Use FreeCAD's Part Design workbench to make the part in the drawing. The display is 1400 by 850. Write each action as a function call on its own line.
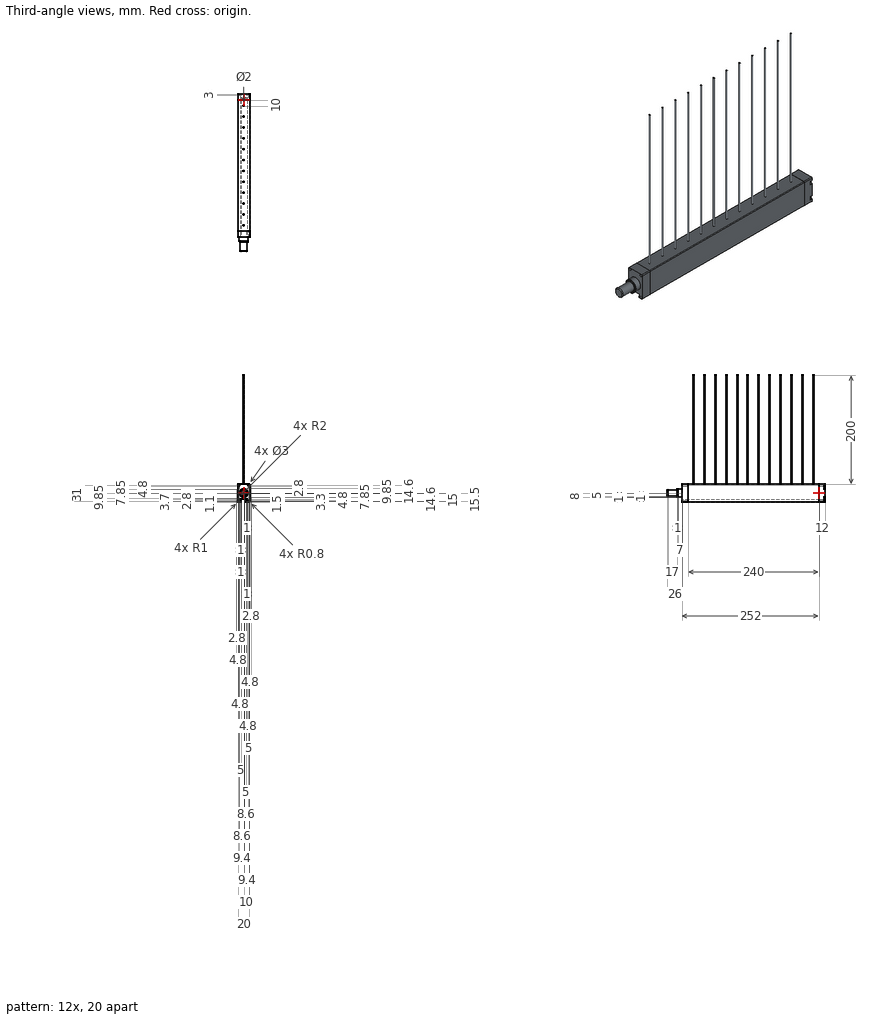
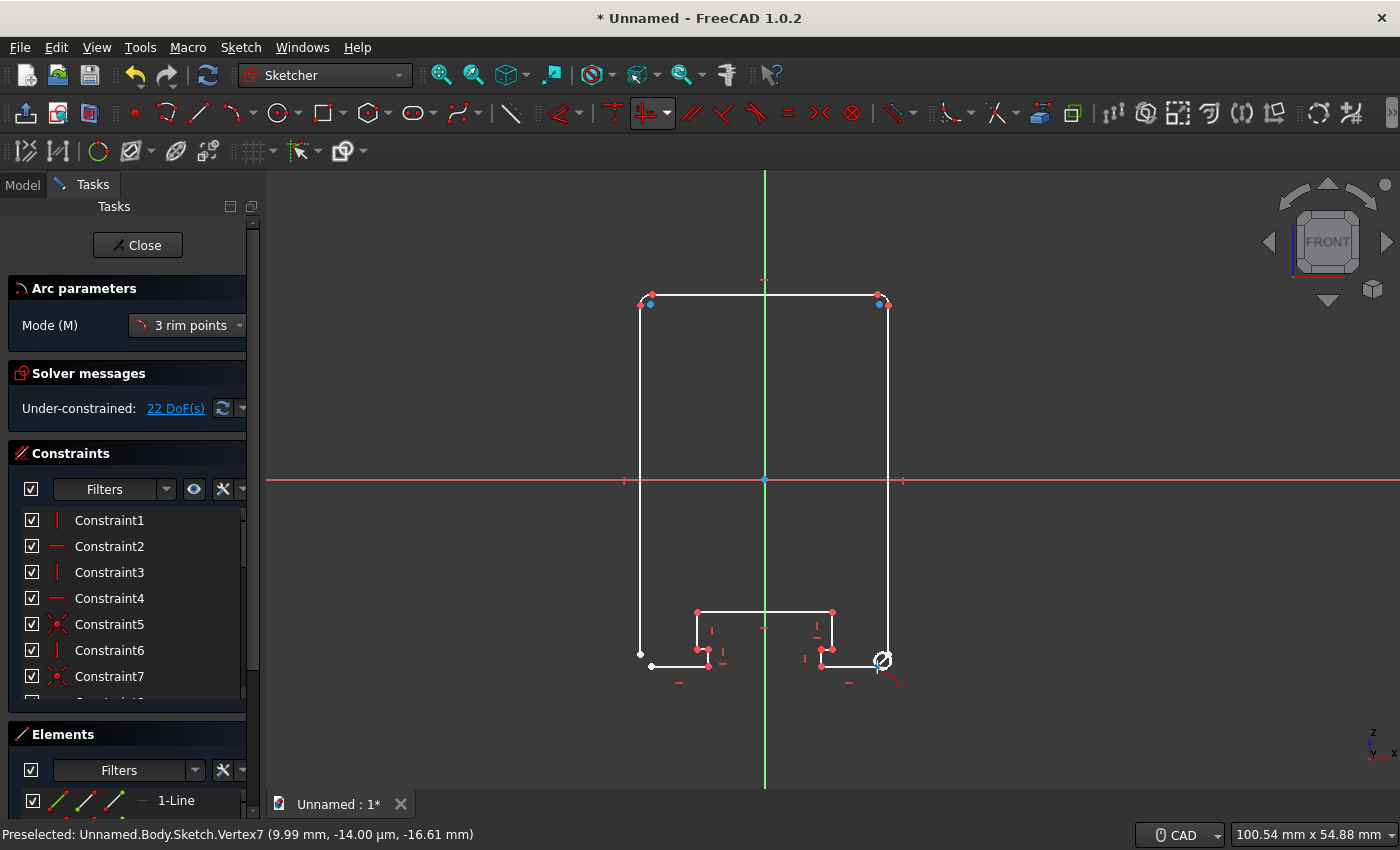
scroll(885, 662, up, 8)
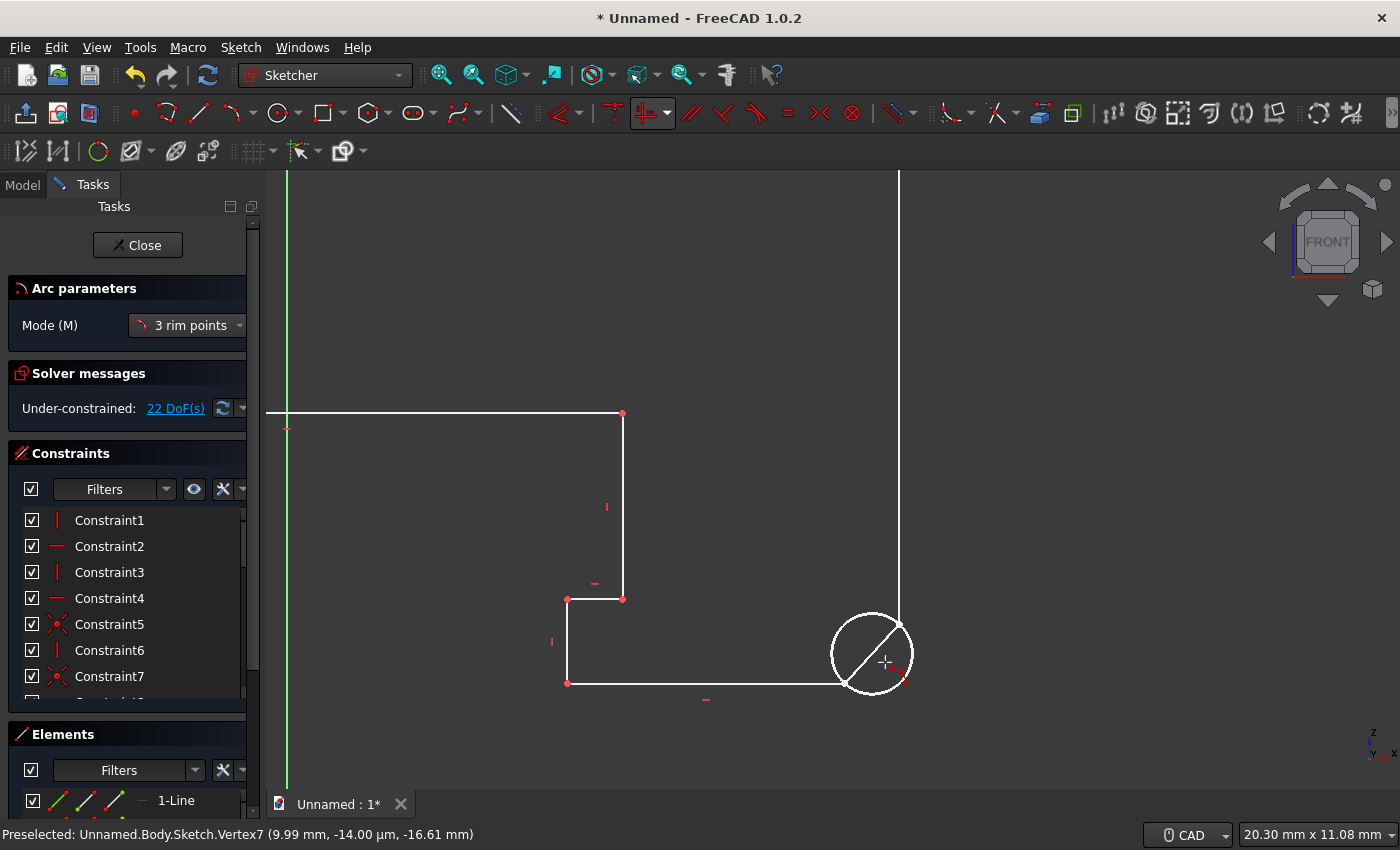
click(885, 661)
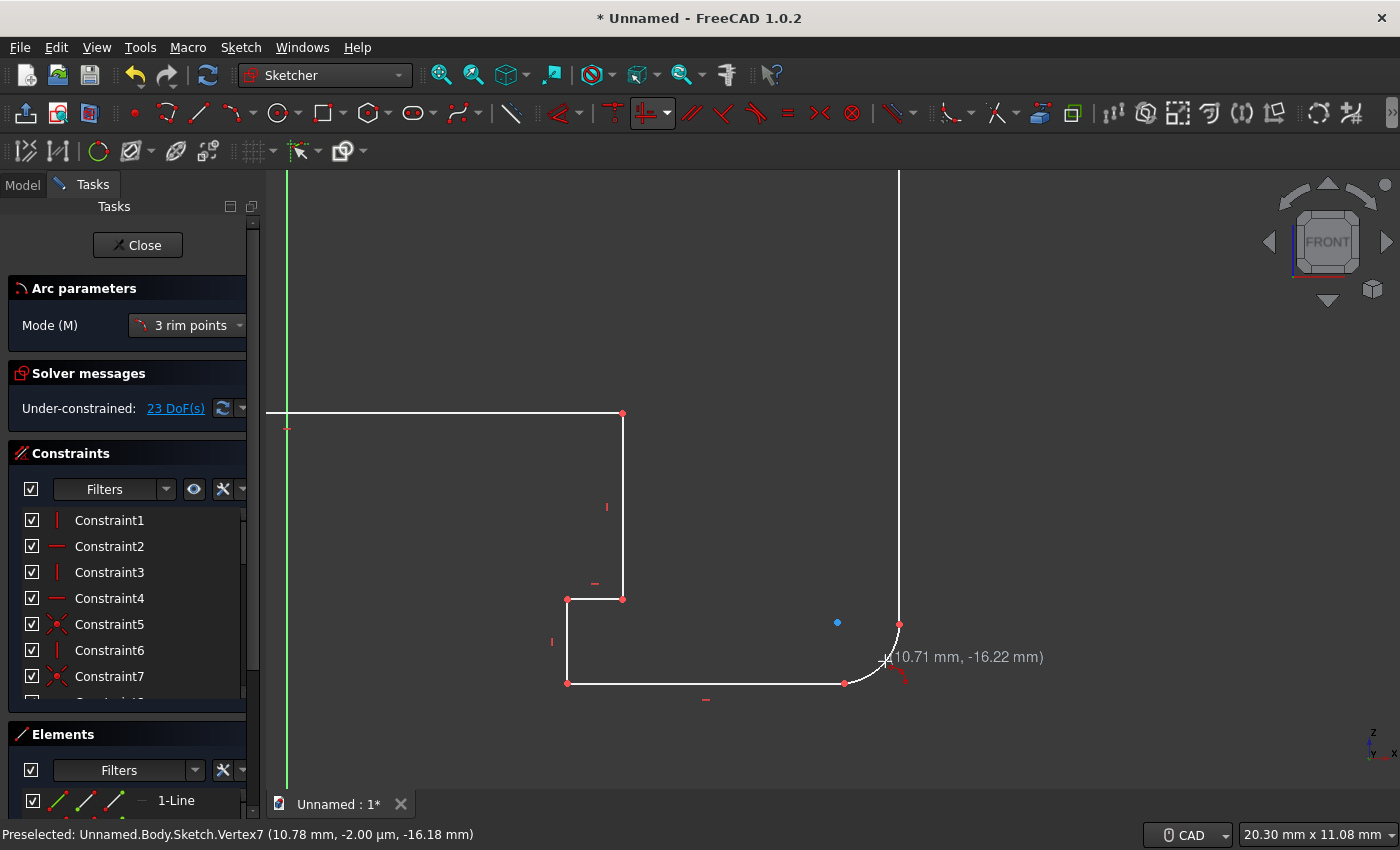
scroll(885, 663, down, 8)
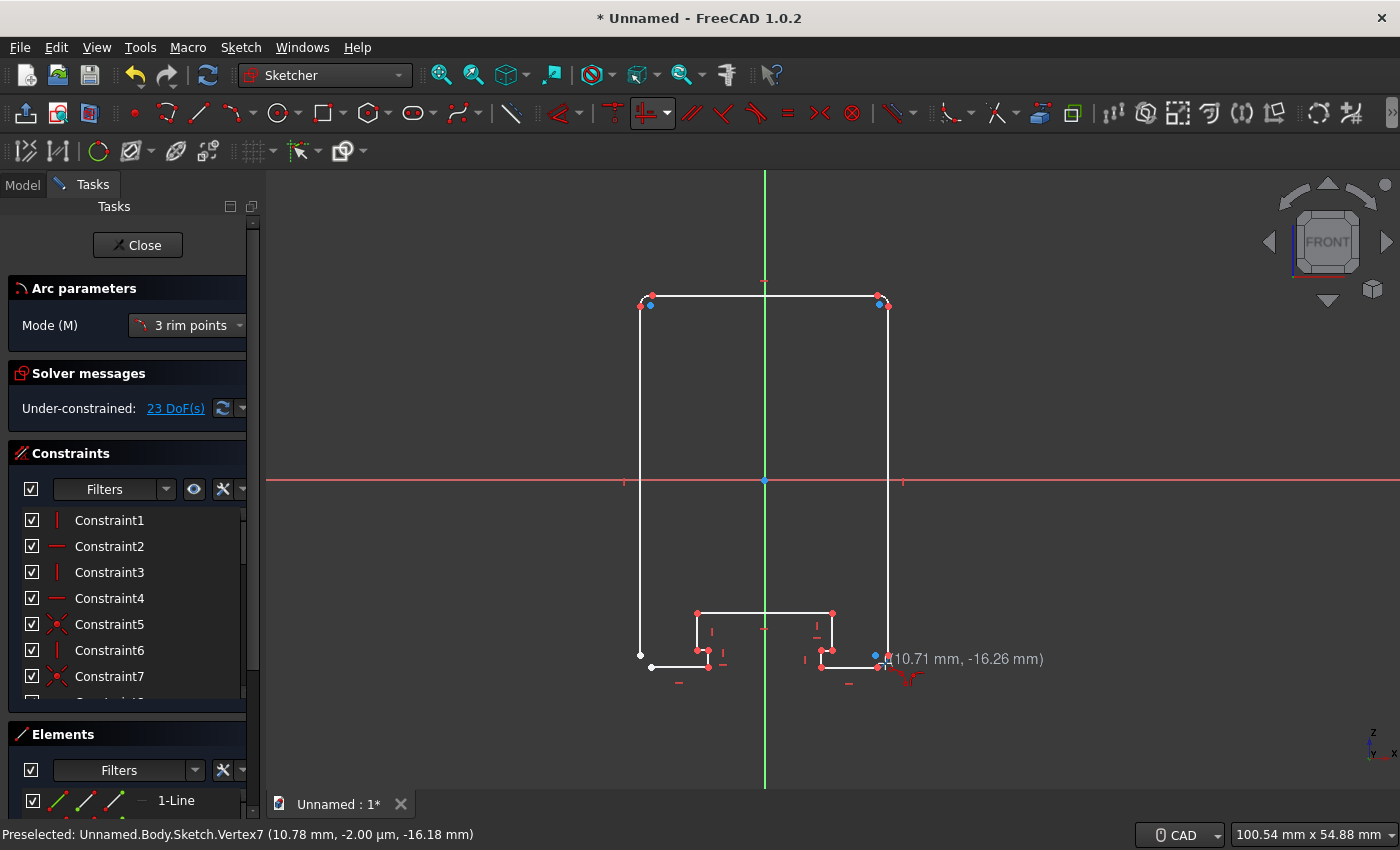
click(652, 667)
click(640, 656)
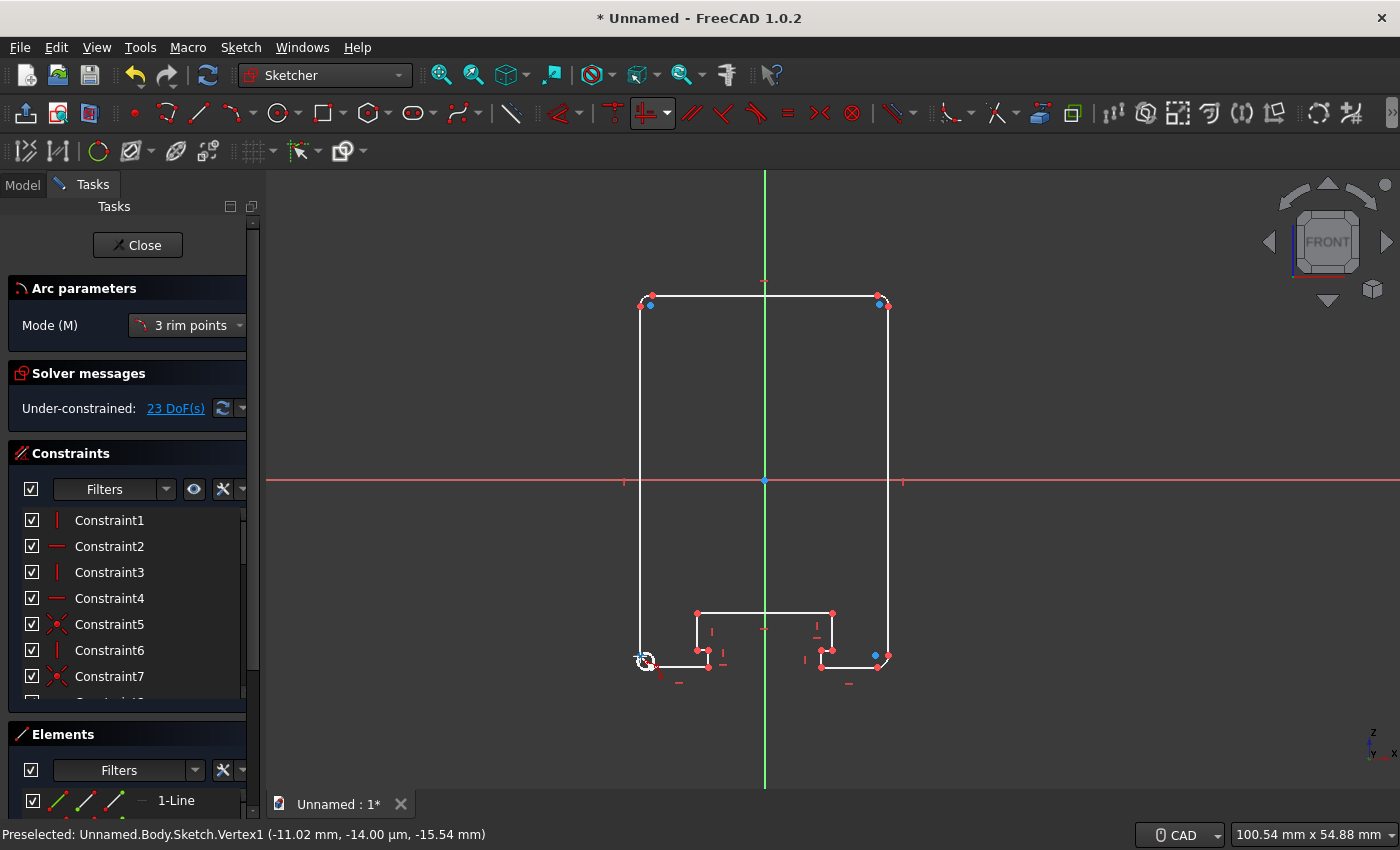
scroll(644, 663, up, 8)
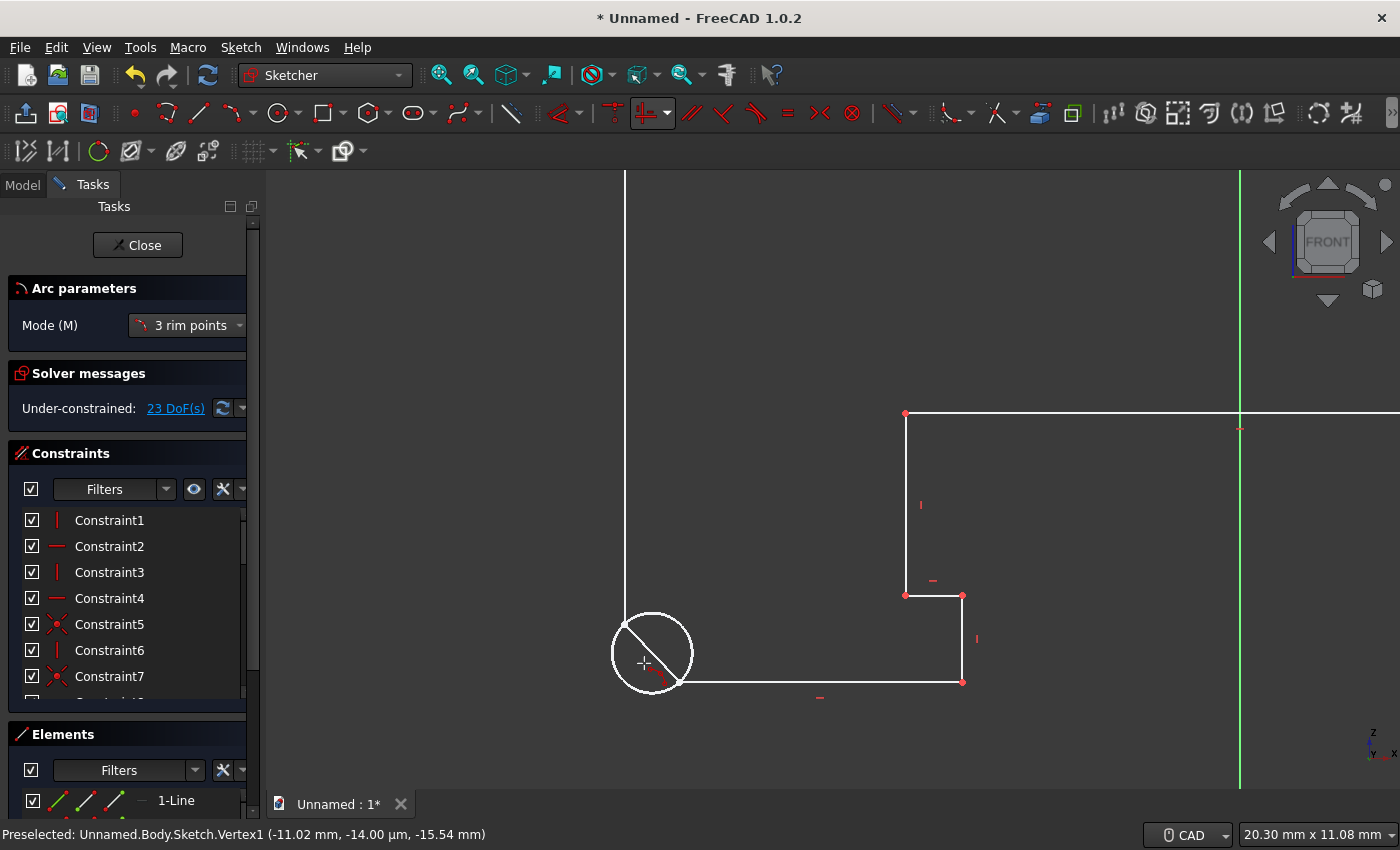
click(642, 661)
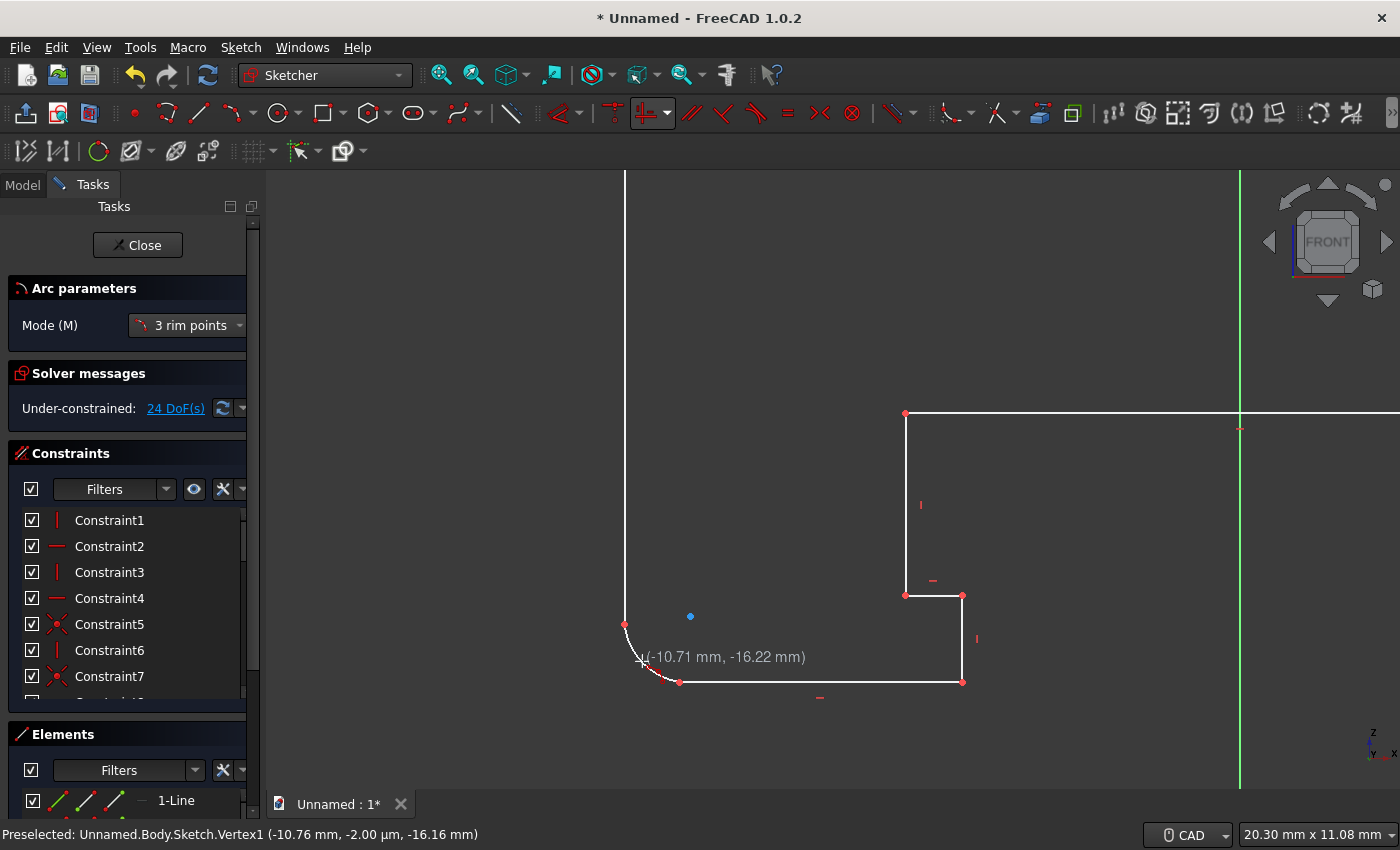
key(g)
key(c)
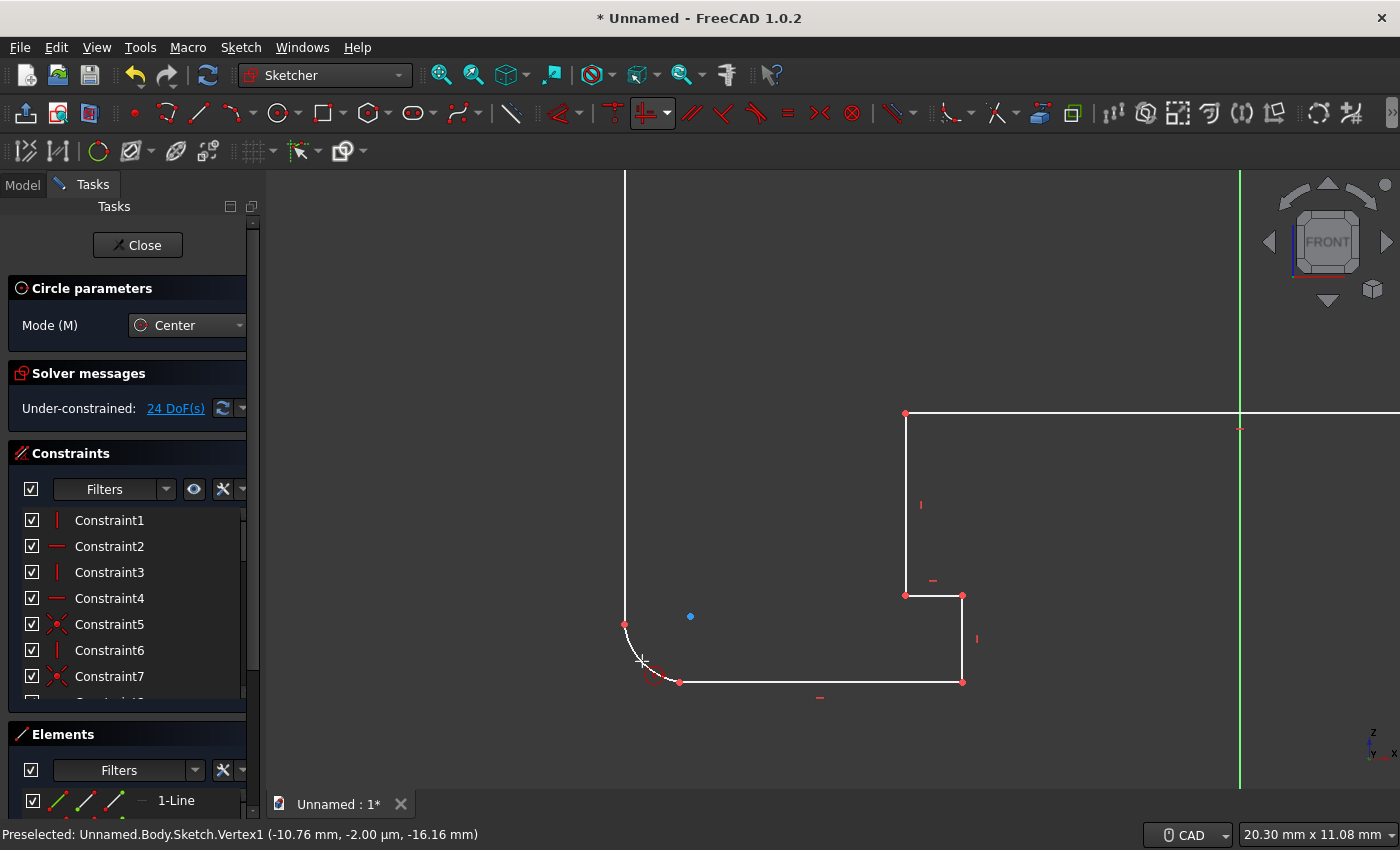
scroll(644, 663, down, 8)